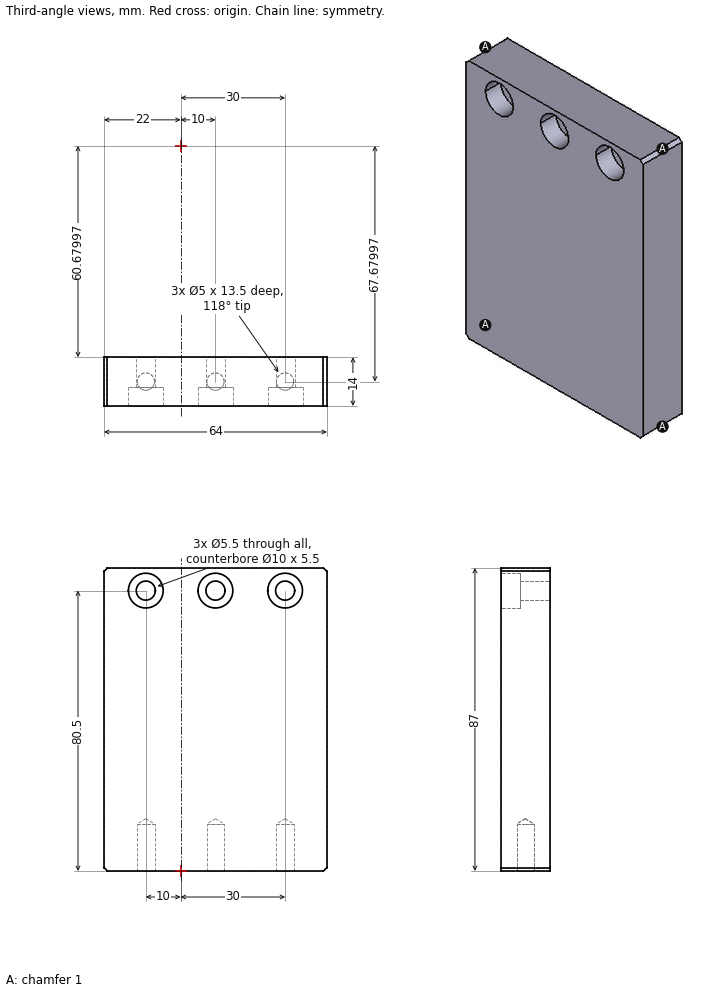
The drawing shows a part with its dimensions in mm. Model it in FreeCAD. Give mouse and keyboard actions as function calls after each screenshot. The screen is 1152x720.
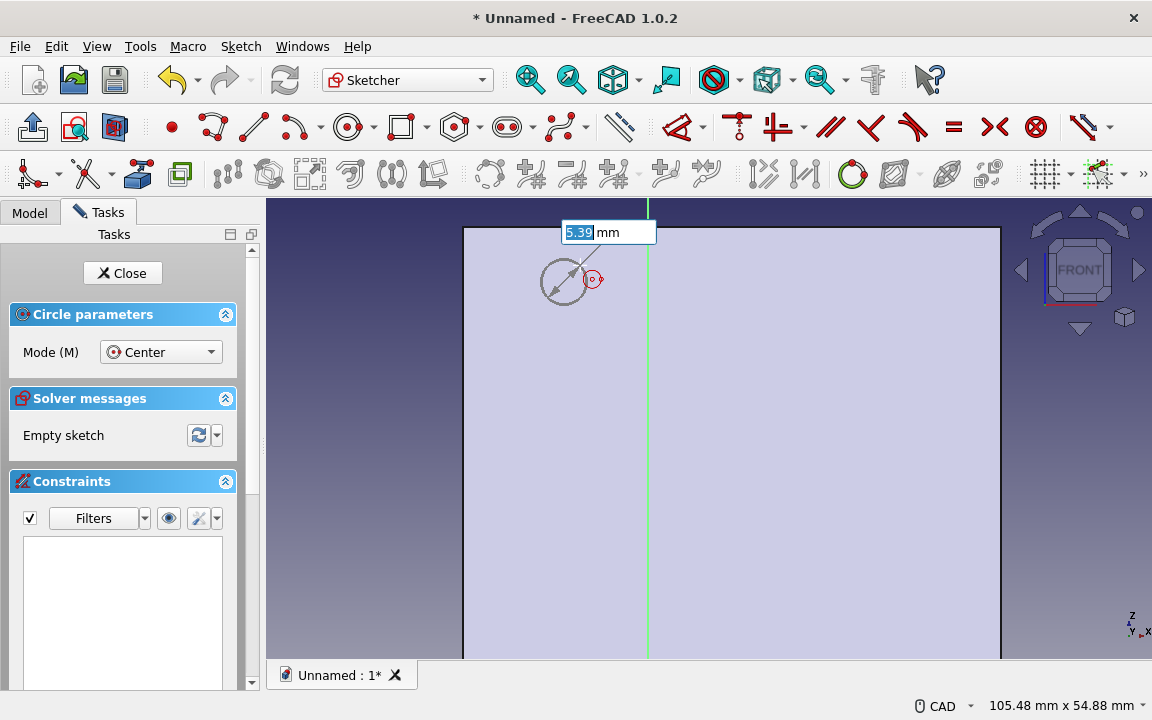
text(5.5)
key(Return)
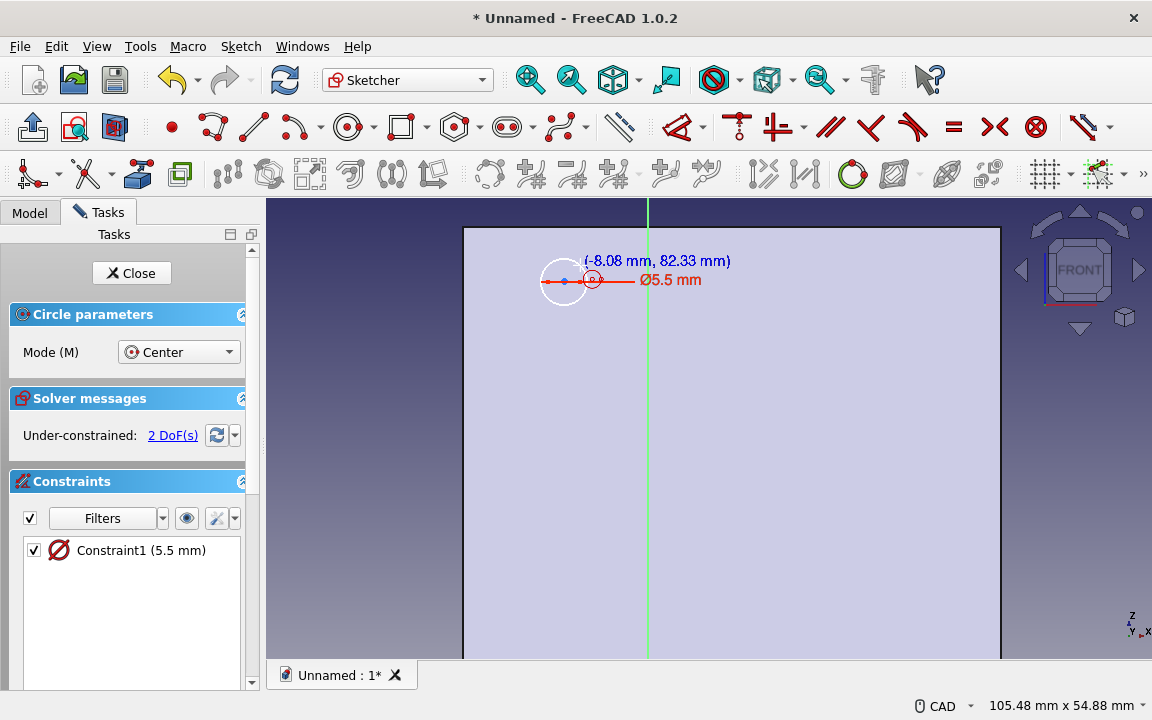
click(732, 281)
move(748, 265)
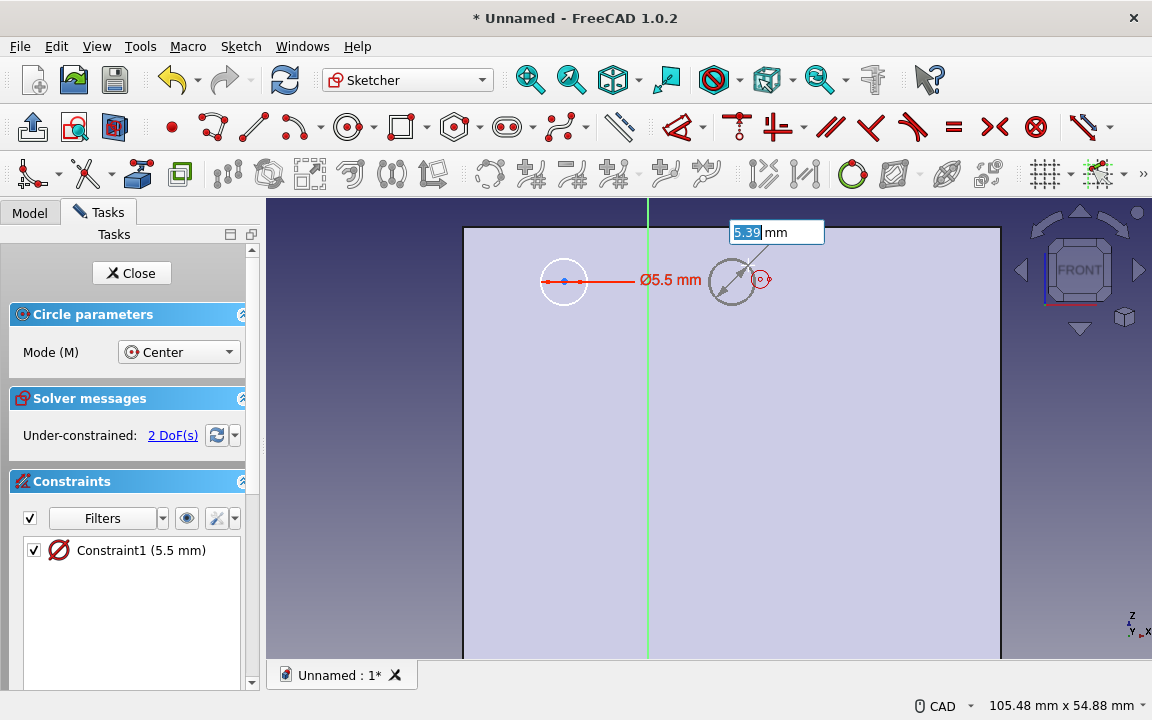
text(5.5)
key(Return)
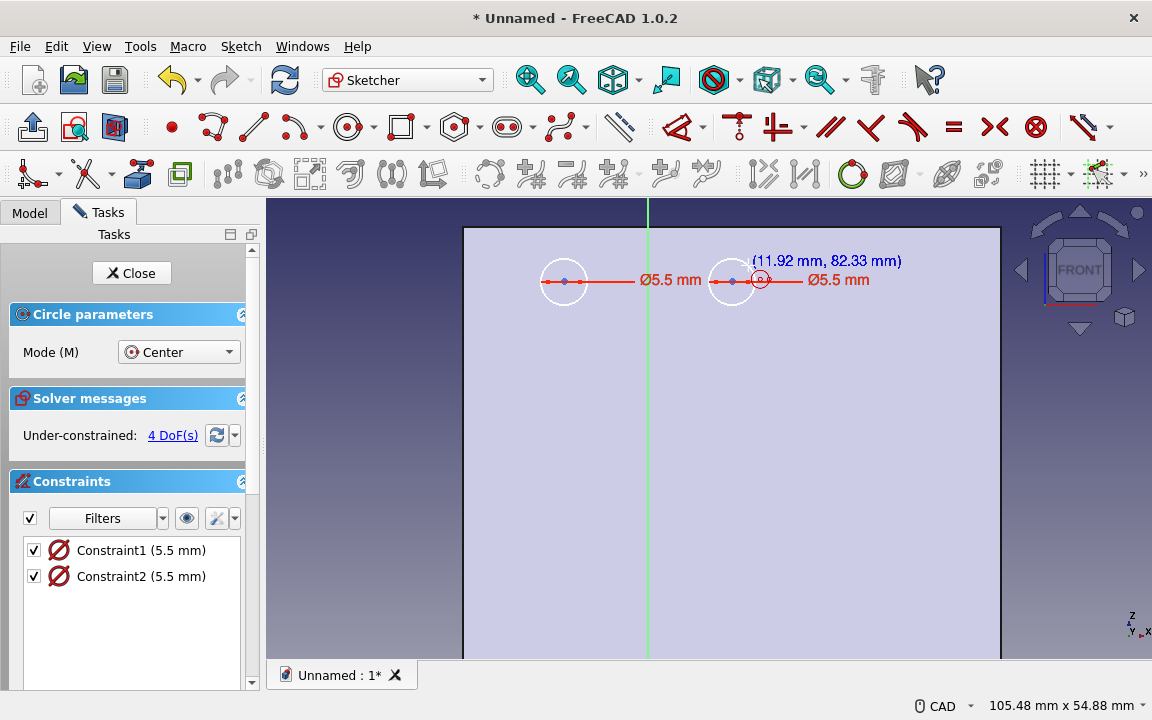
click(900, 281)
move(916, 265)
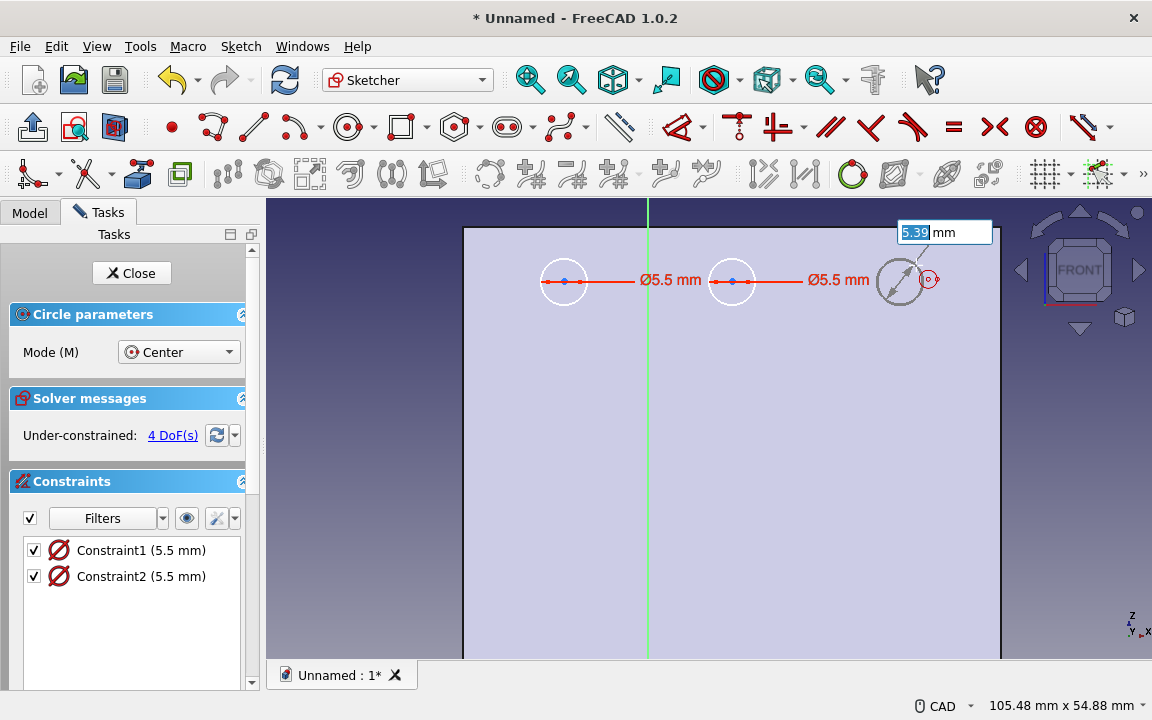
text(5.5)
key(Return)
key(Escape)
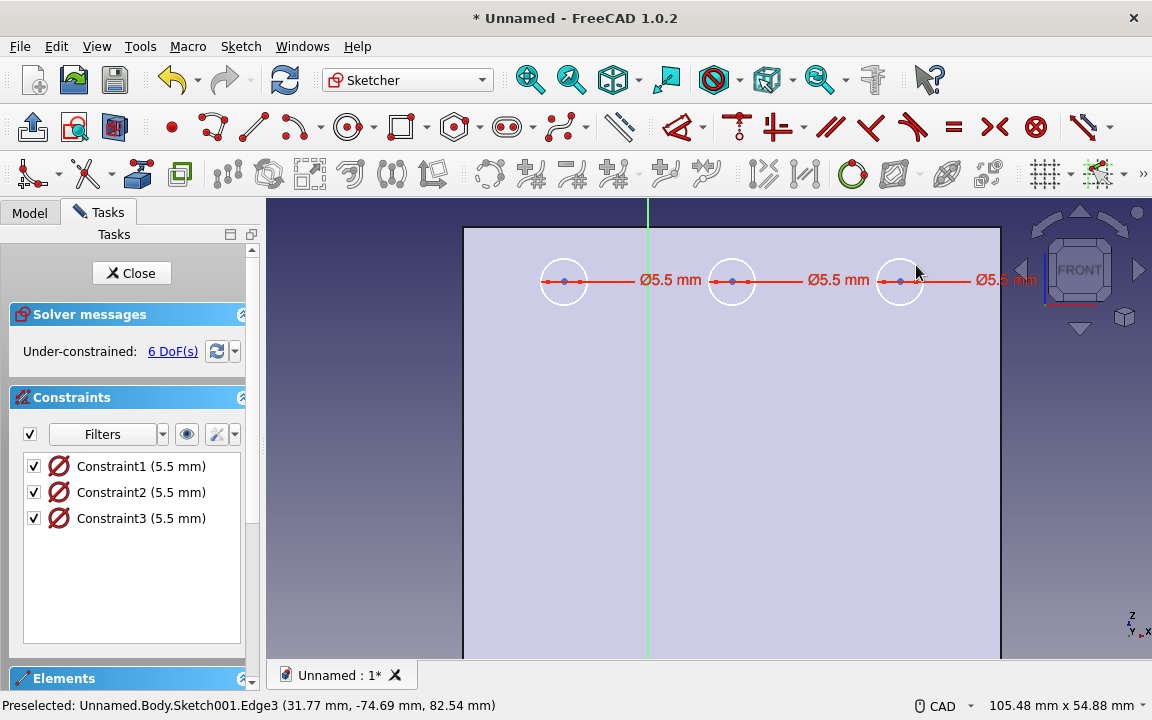
click(564, 282)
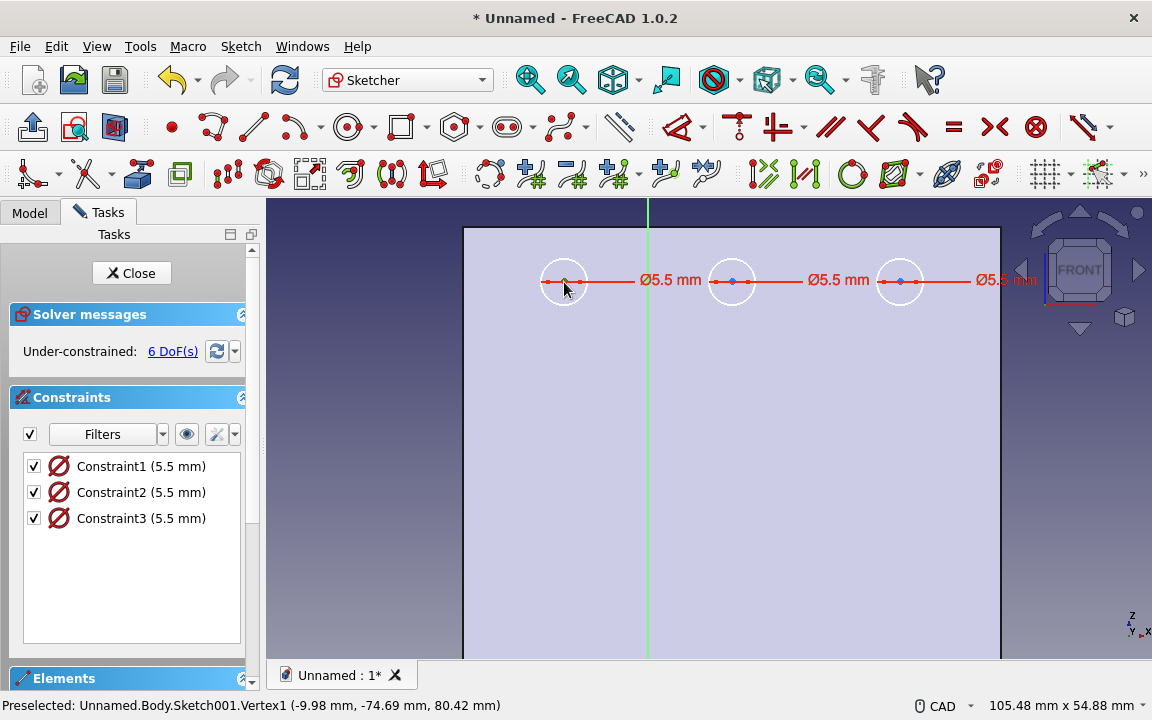
click(732, 282)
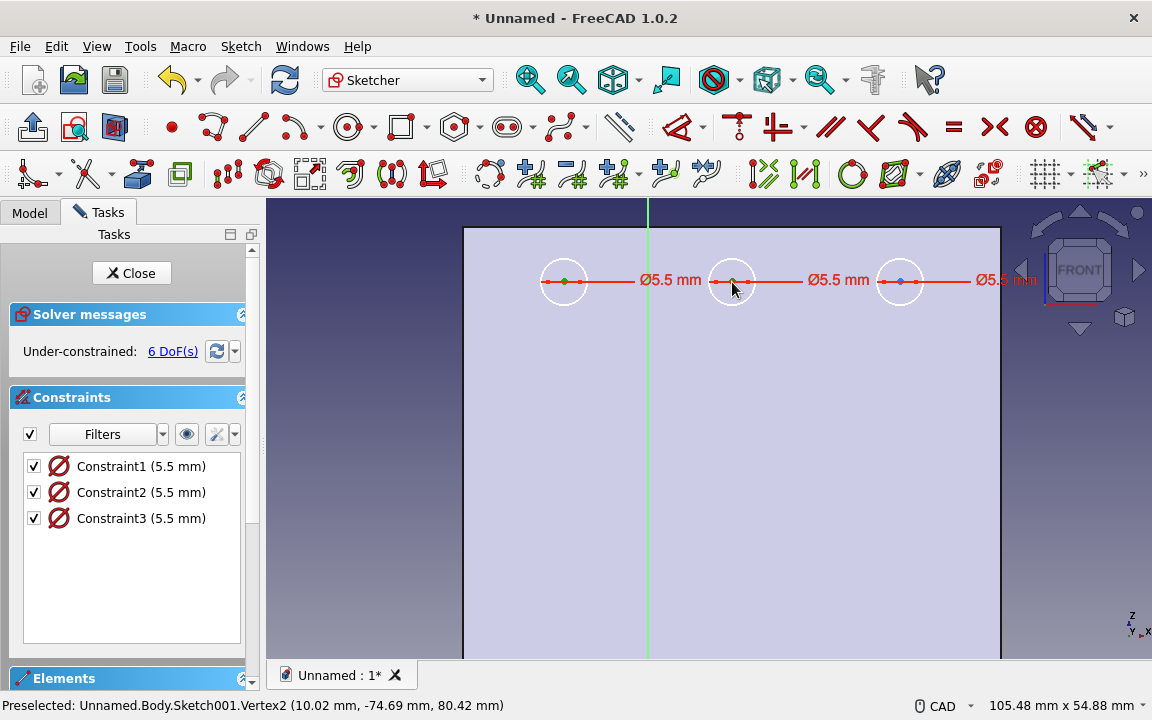
click(648, 602)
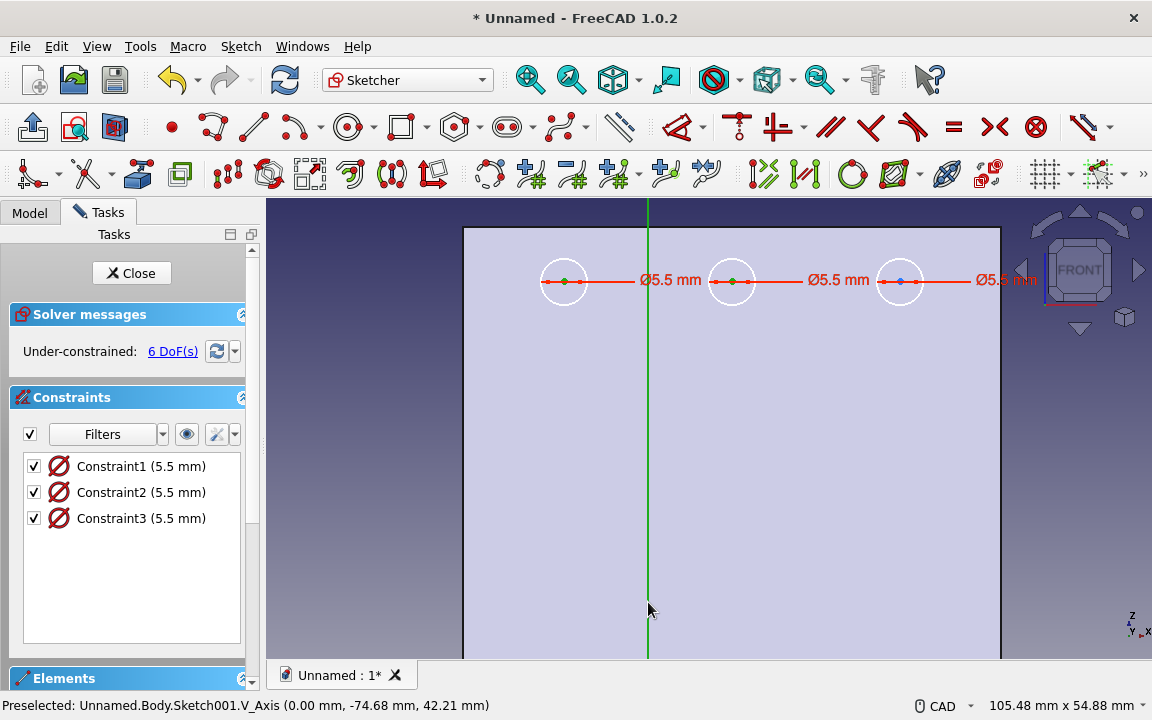
key(s)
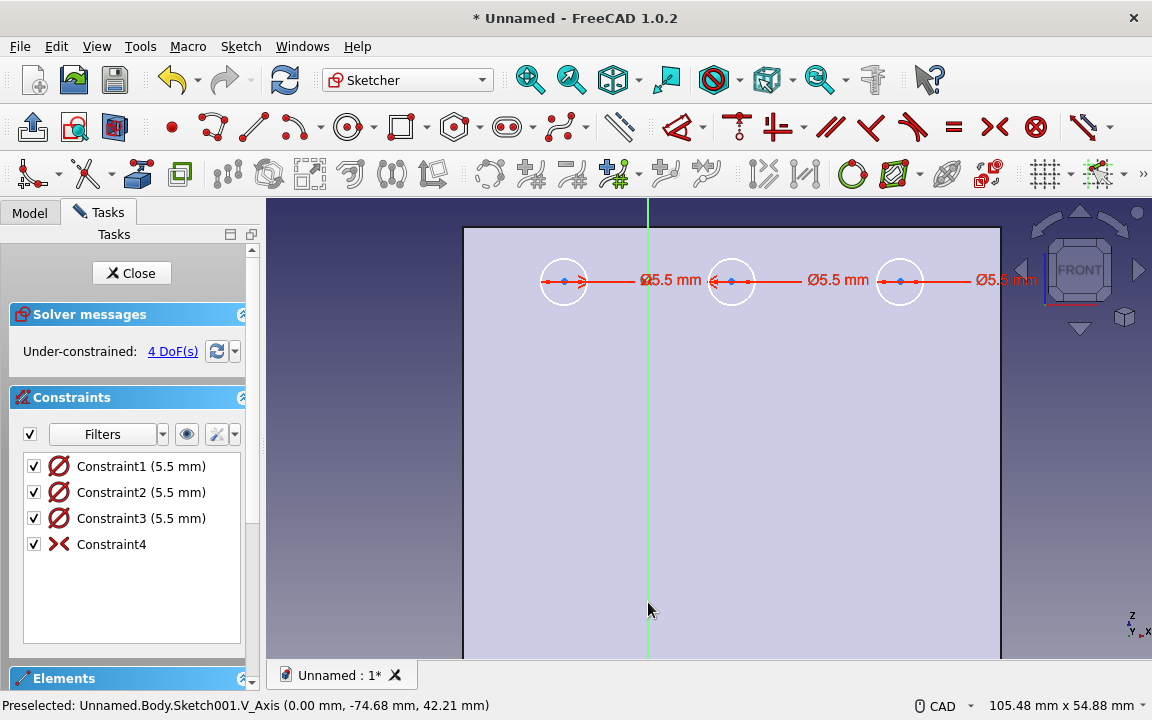
key(d)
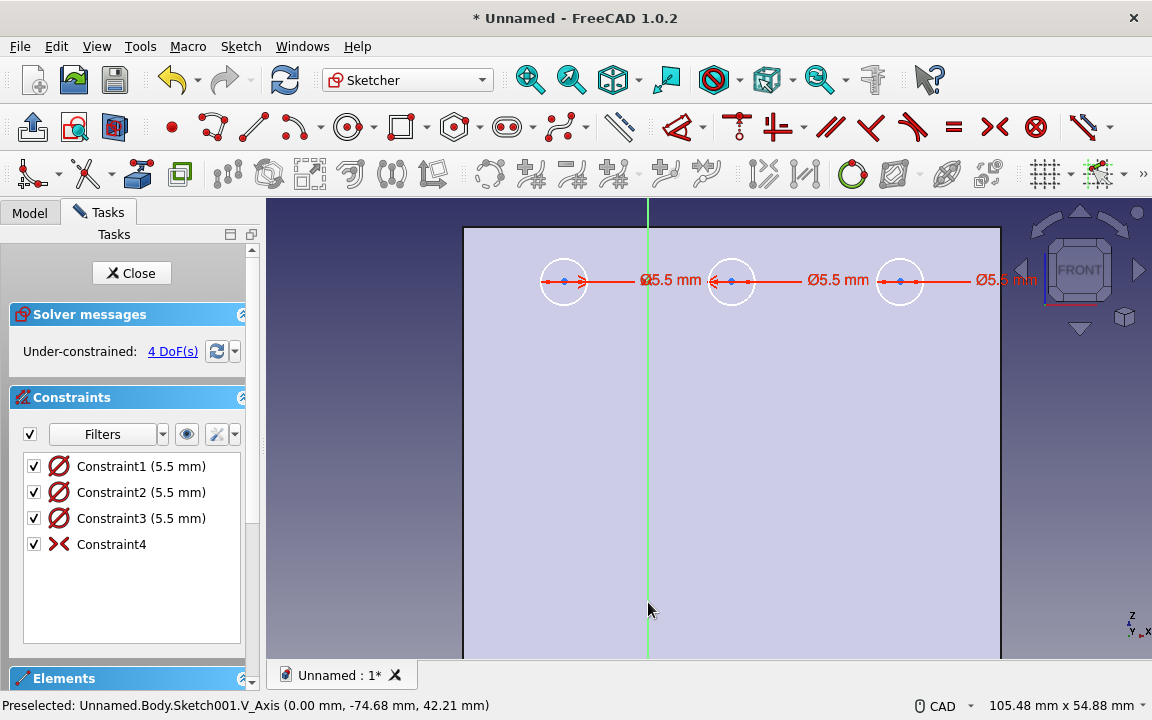
click(564, 282)
click(606, 248)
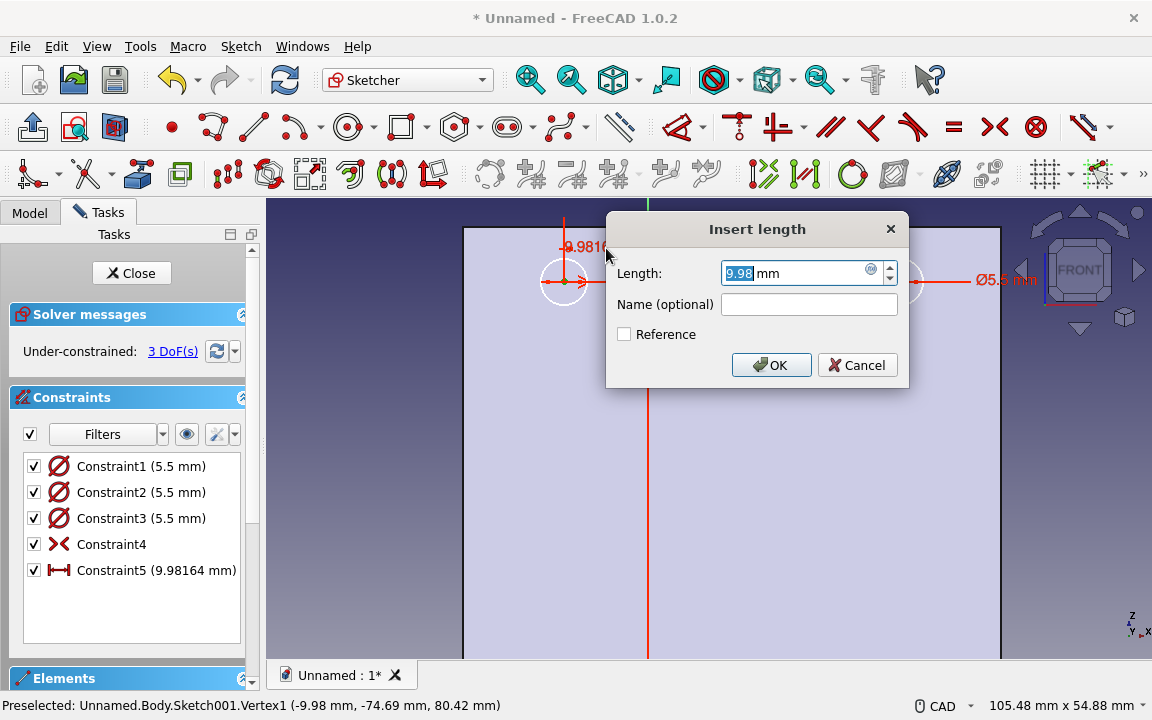
text(10)
key(Return)